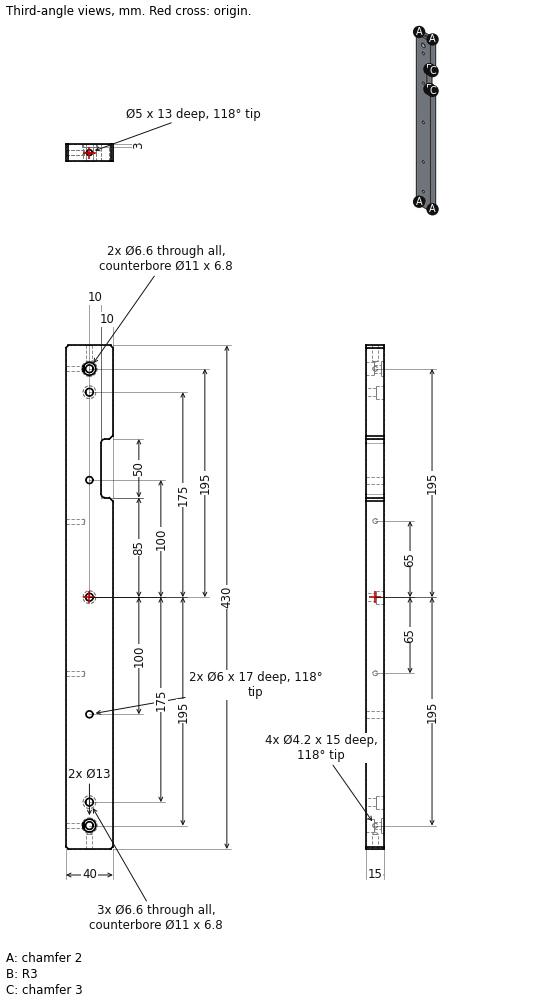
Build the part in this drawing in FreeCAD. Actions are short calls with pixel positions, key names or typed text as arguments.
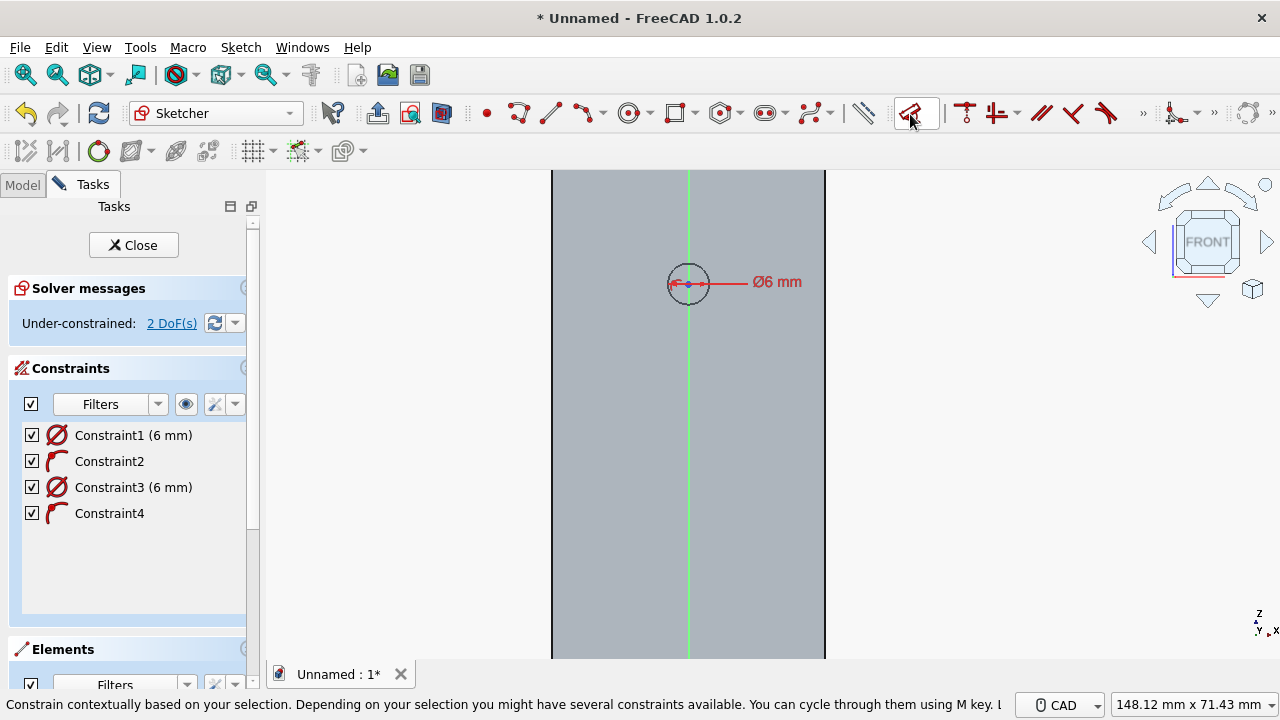
scroll(709, 275, down, 8)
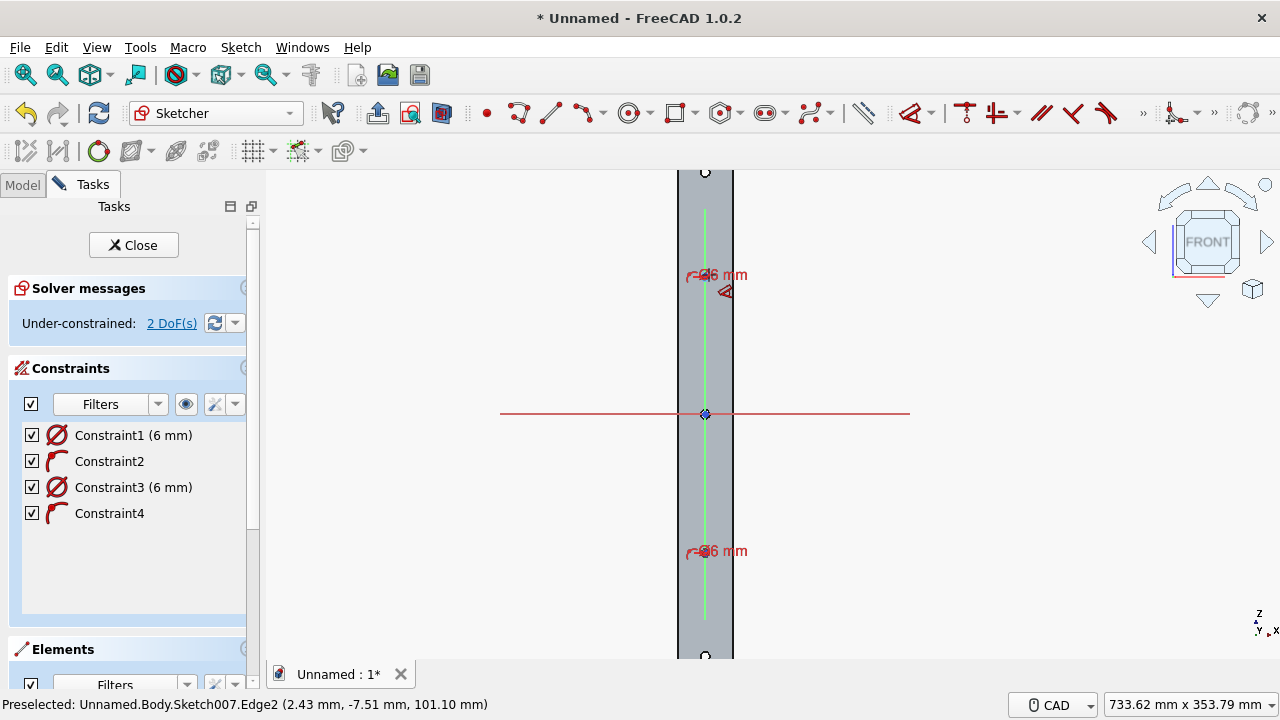
click(705, 553)
click(739, 484)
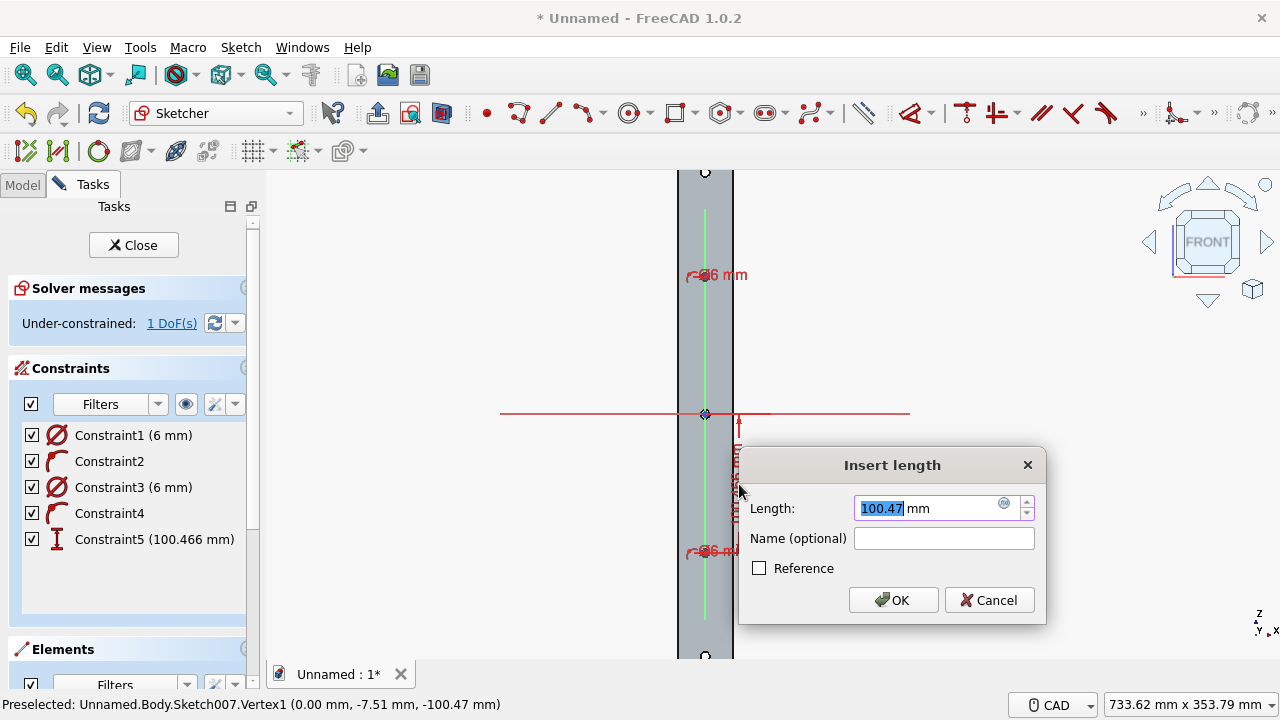
text(100)
key(Return)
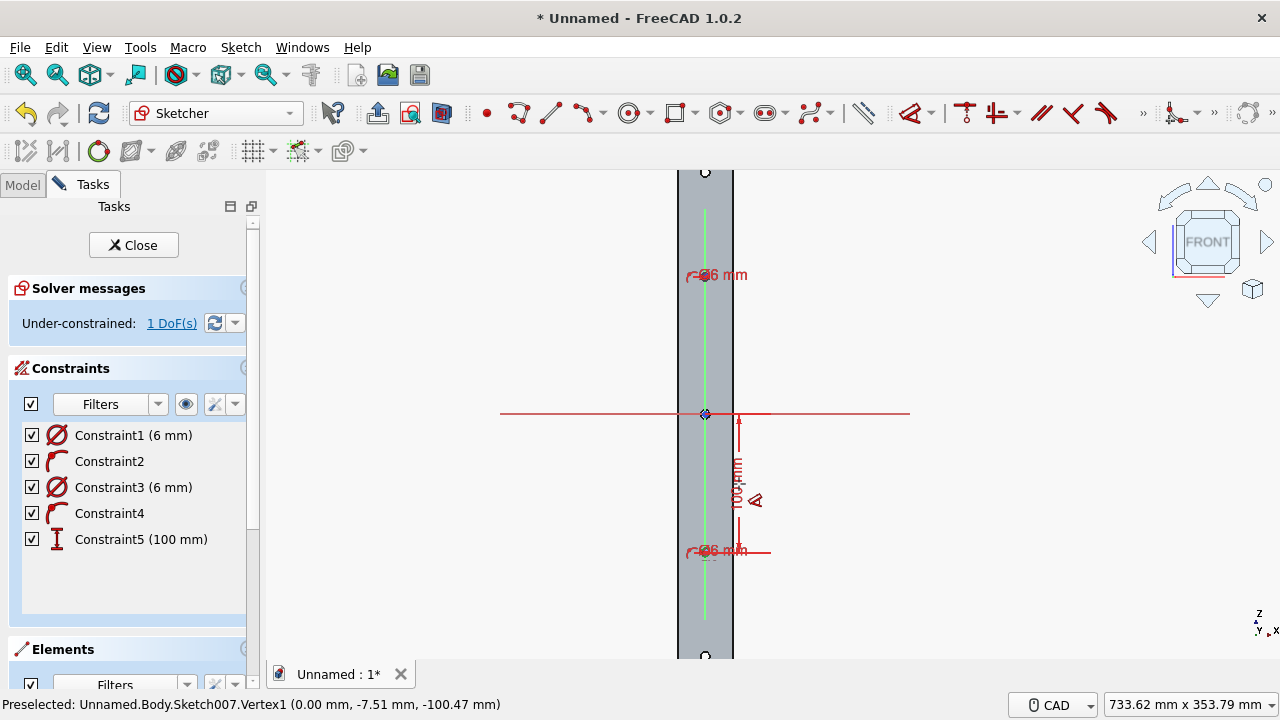
click(705, 277)
click(739, 346)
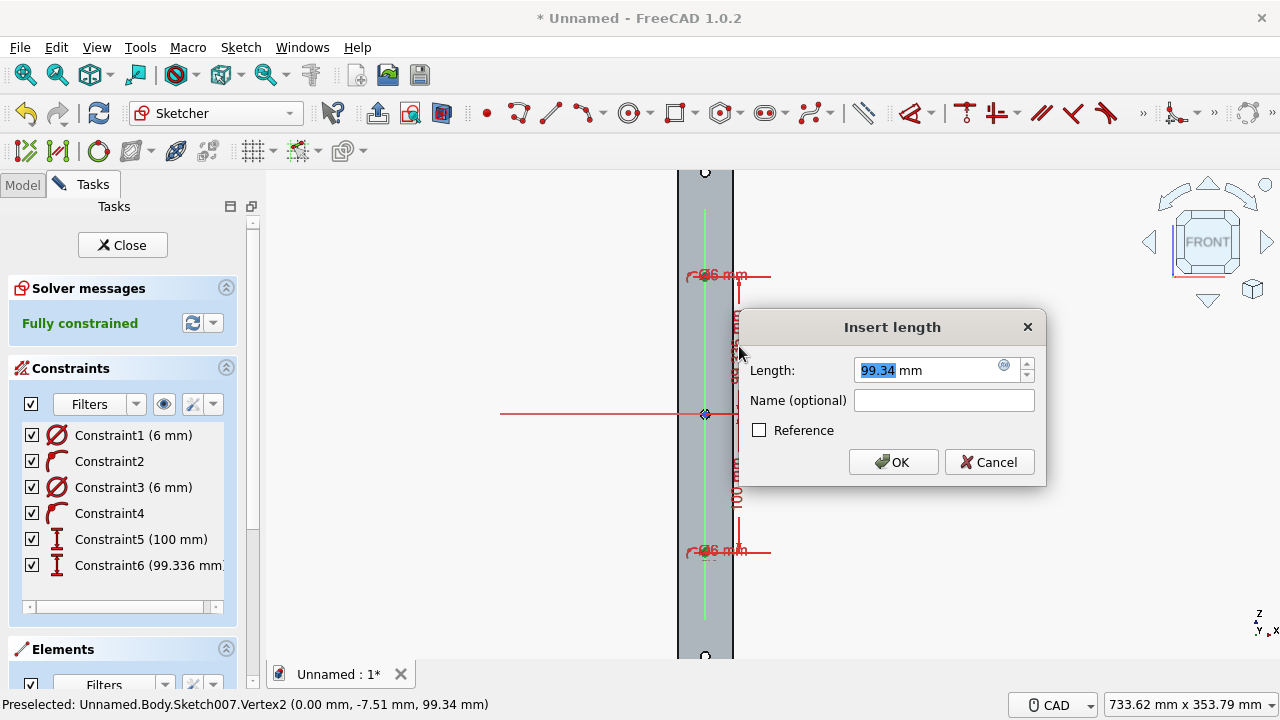
text(100)
key(Return)
key(Escape)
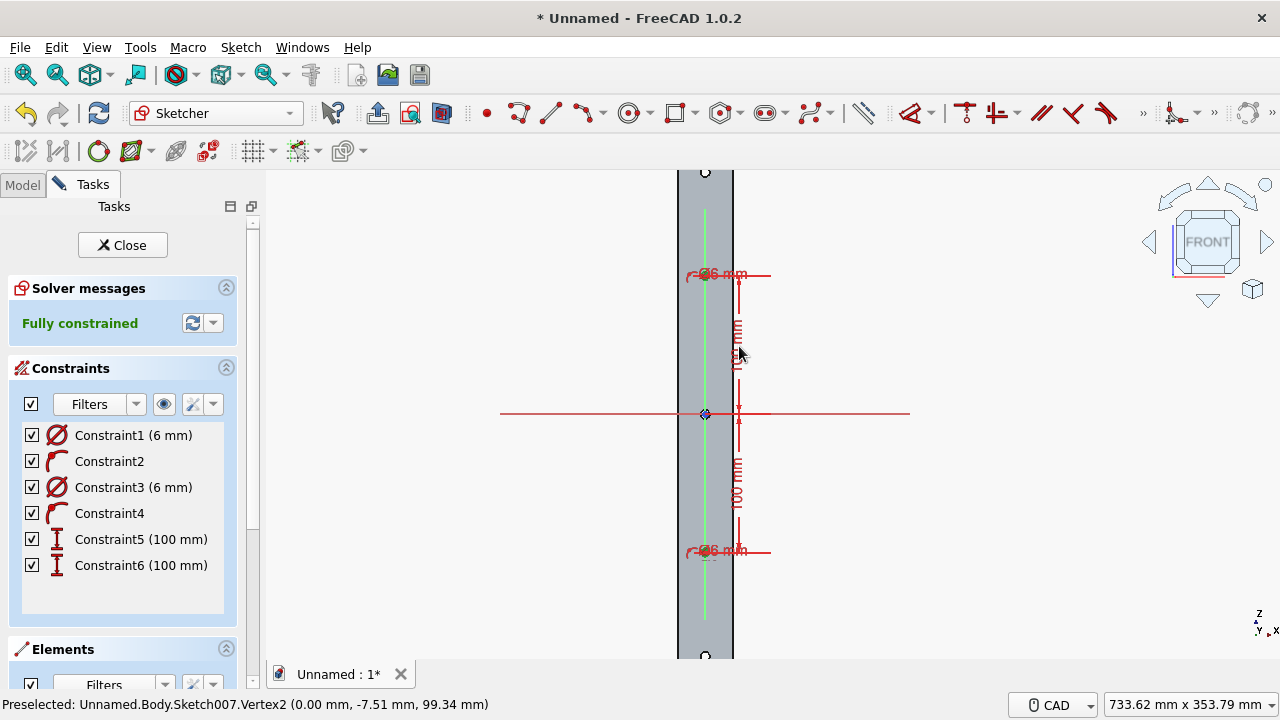
click(123, 245)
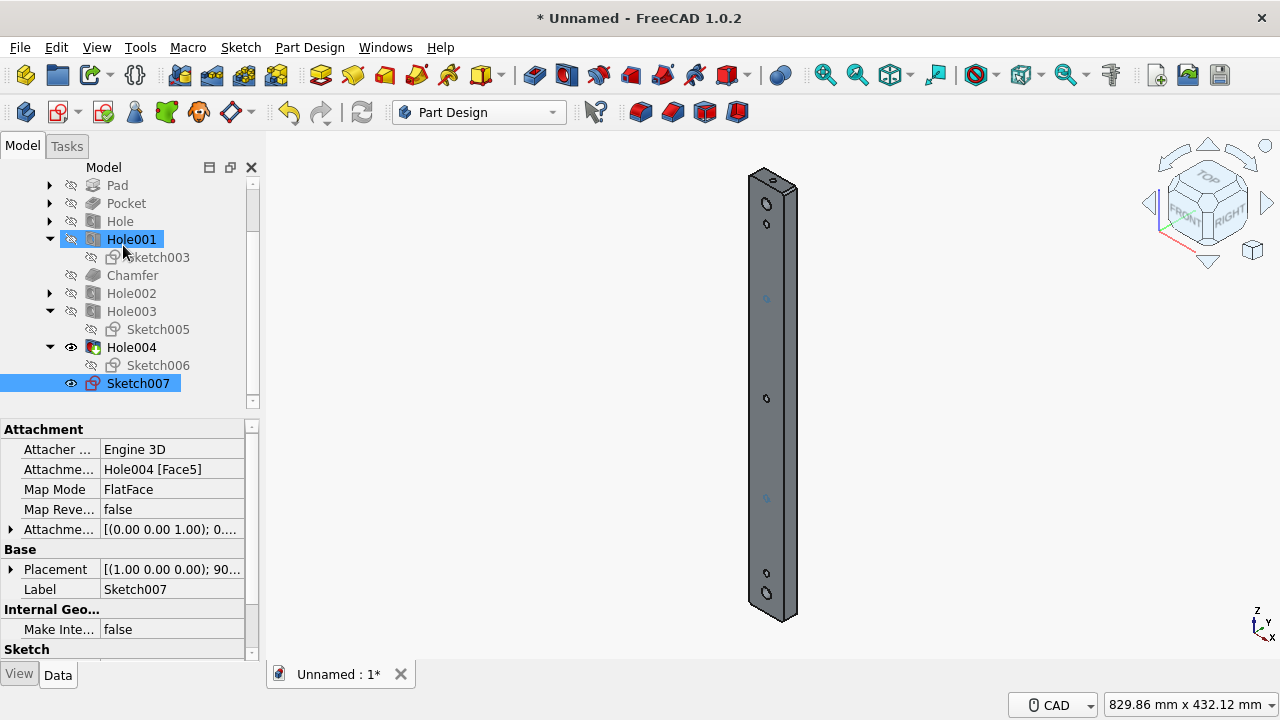
click(568, 76)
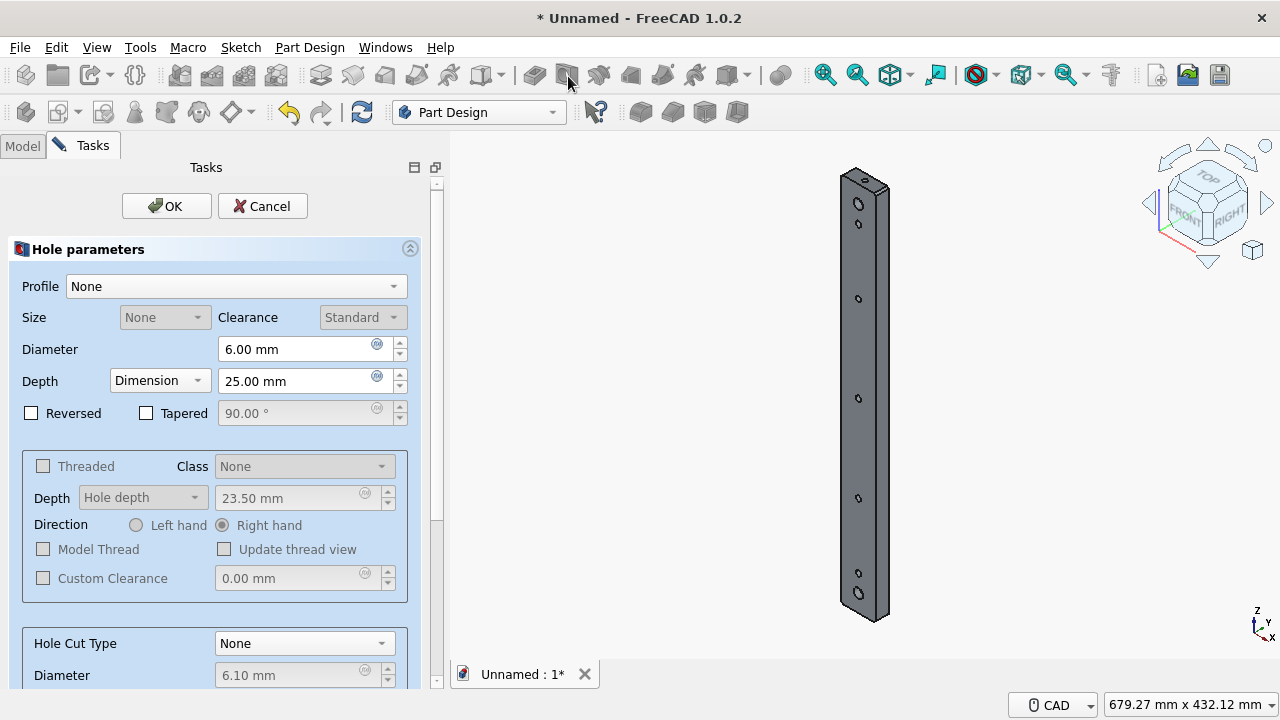
triple_click(305, 349)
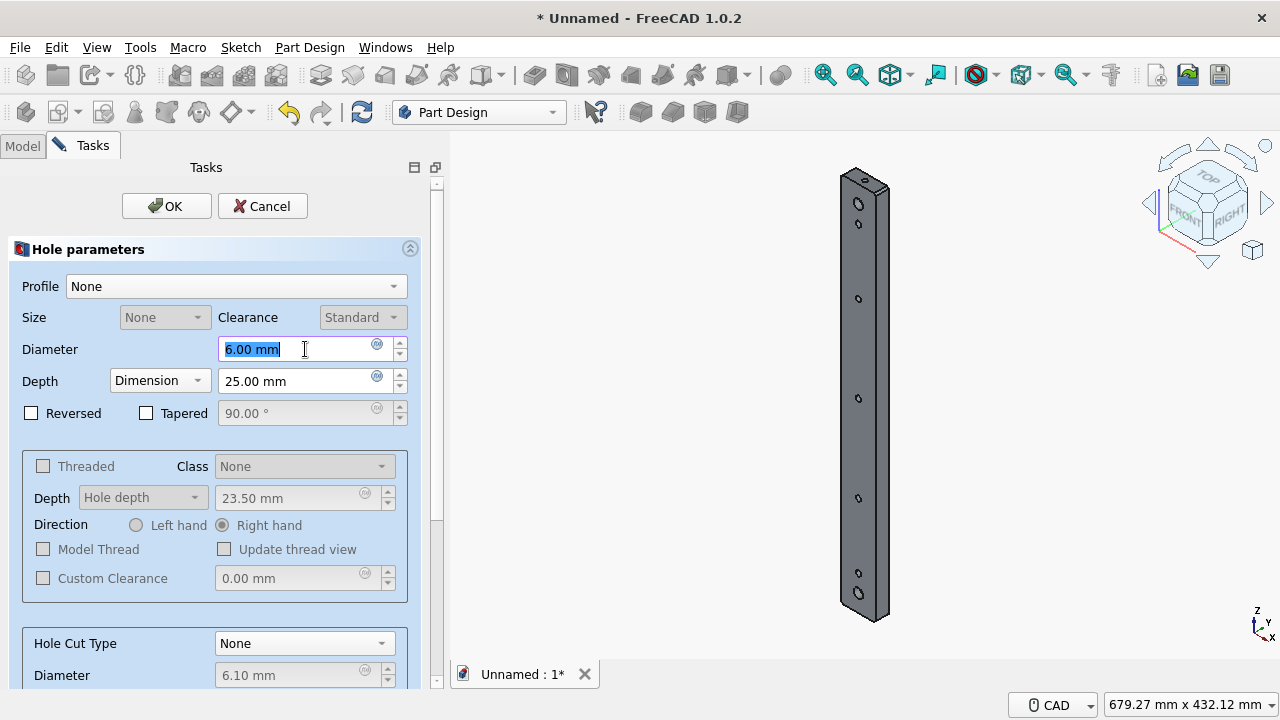
text(6)
key(Tab)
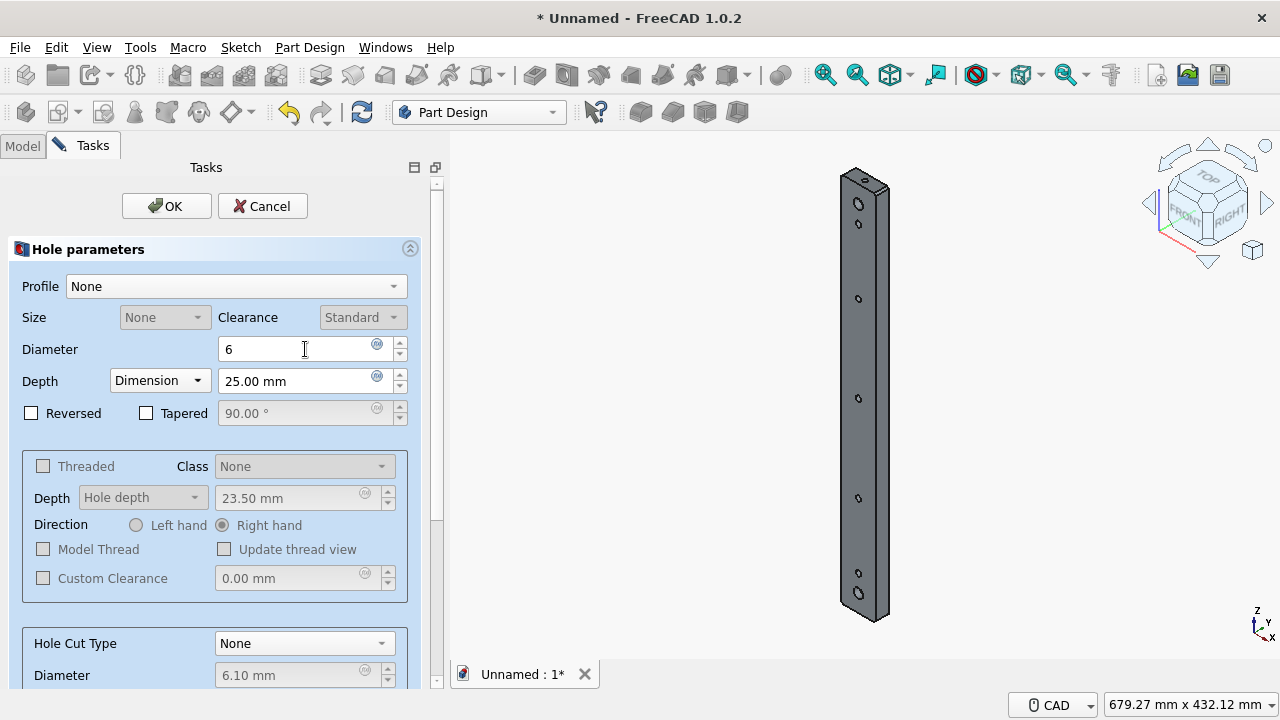
triple_click(305, 381)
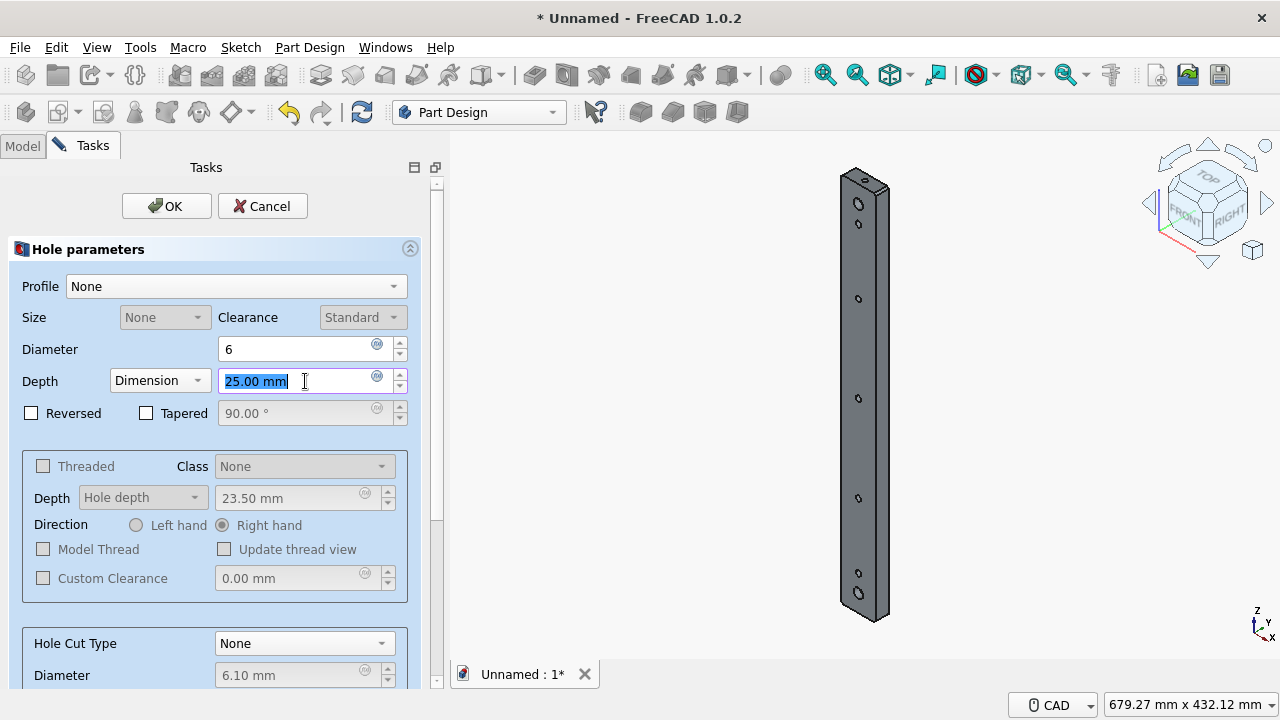
text(17)
key(Tab)